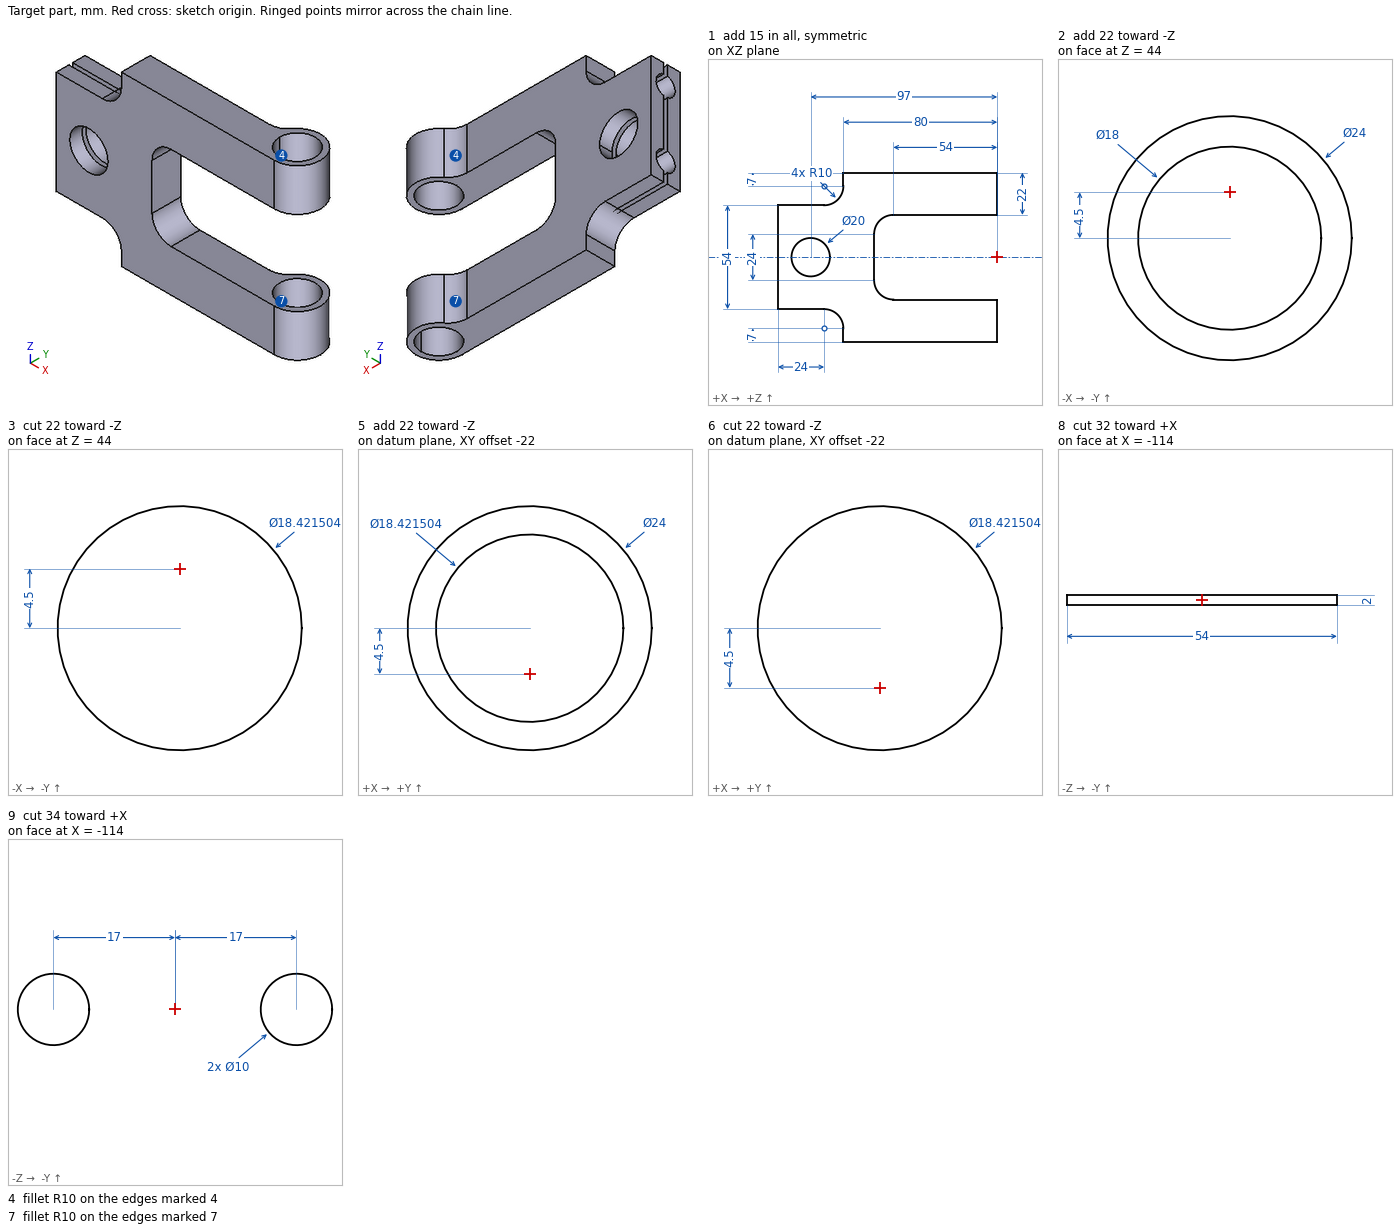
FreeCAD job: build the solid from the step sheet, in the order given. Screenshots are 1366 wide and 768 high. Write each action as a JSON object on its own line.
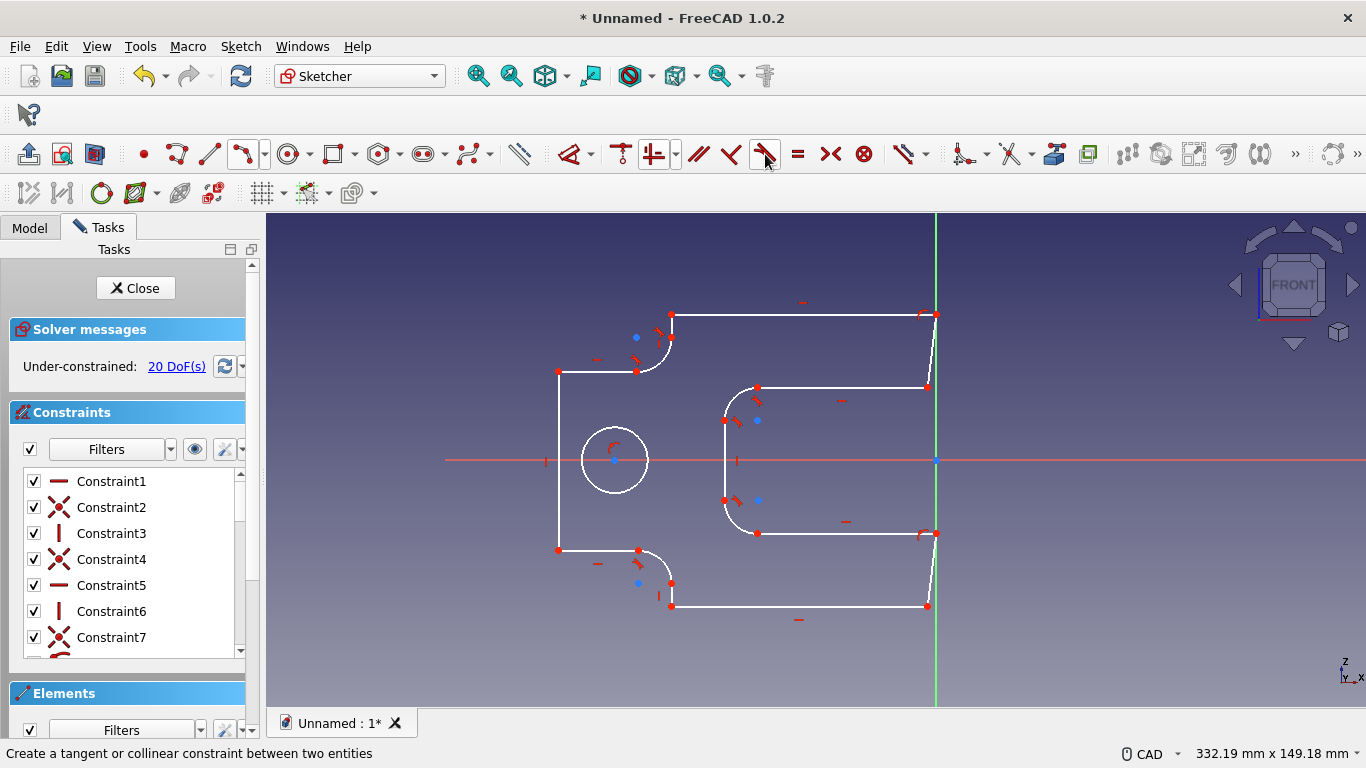
{"action": "left_click", "coordinate": [811, 534]}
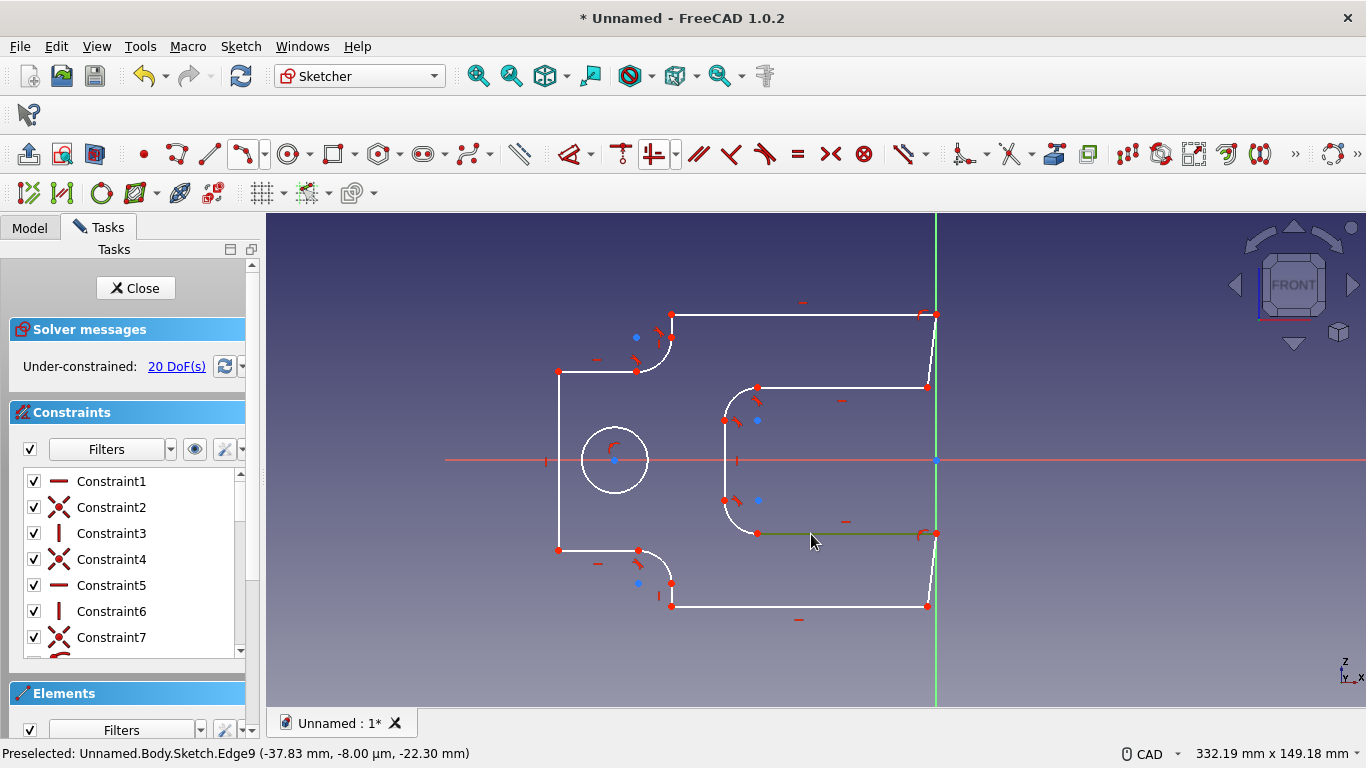
{"action": "left_click", "coordinate": [728, 515]}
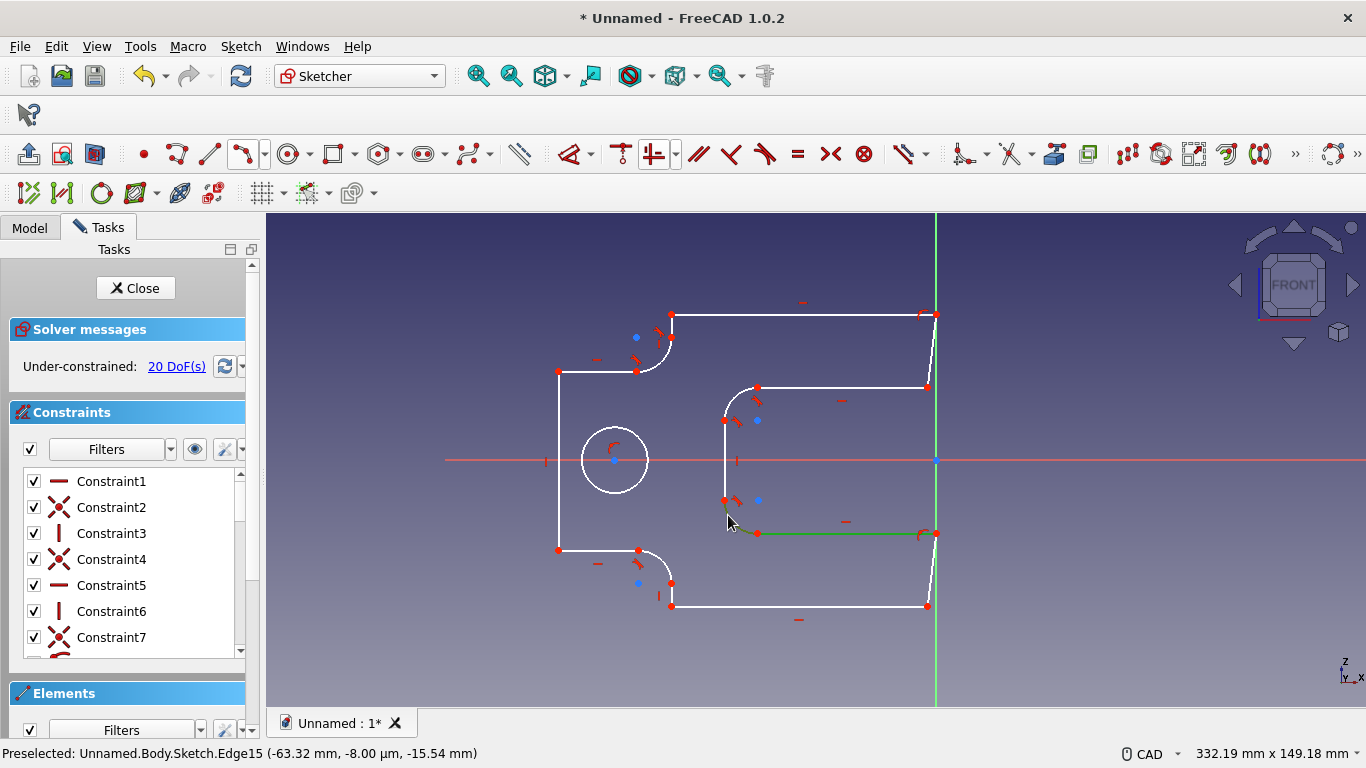
{"action": "left_click", "coordinate": [765, 154]}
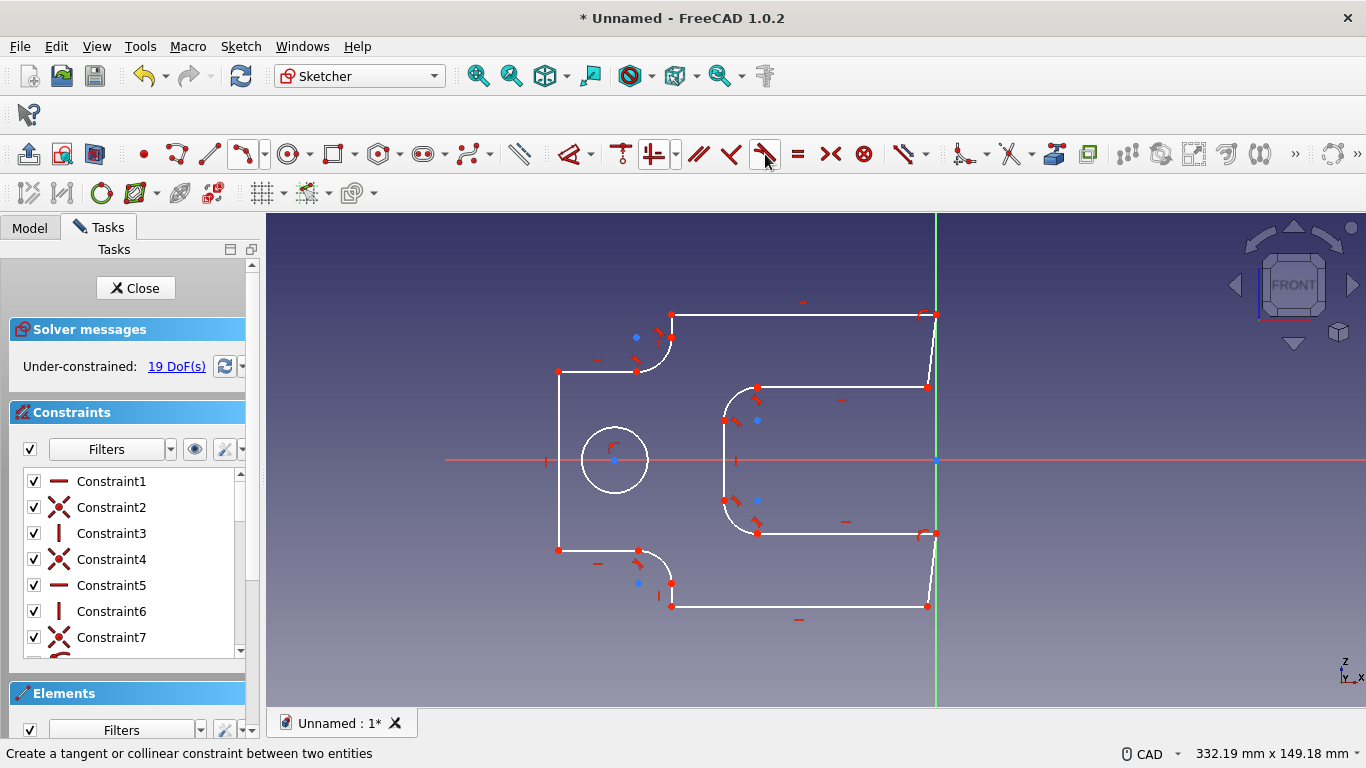
{"action": "scroll", "coordinate": [672, 598], "scroll_direction": "up", "scroll_amount": 3}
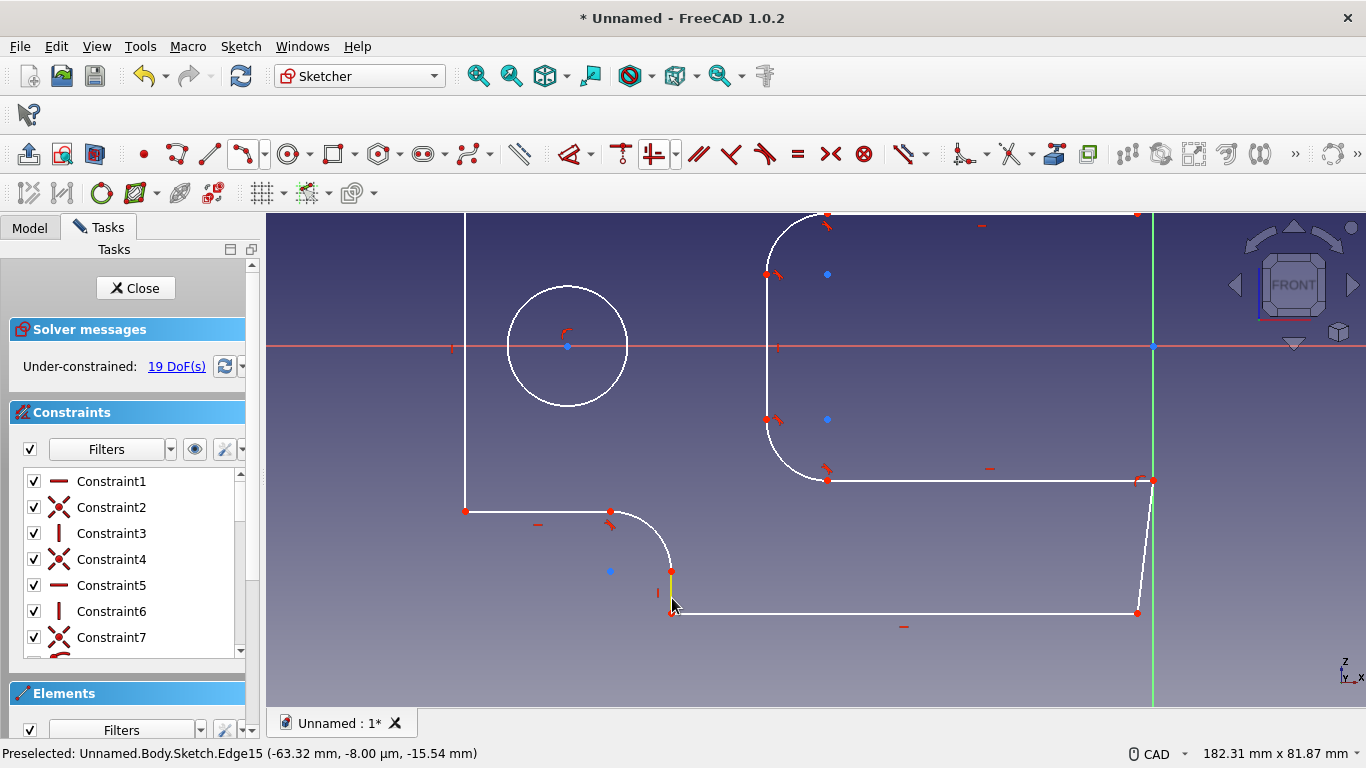
{"action": "left_click", "coordinate": [671, 597]}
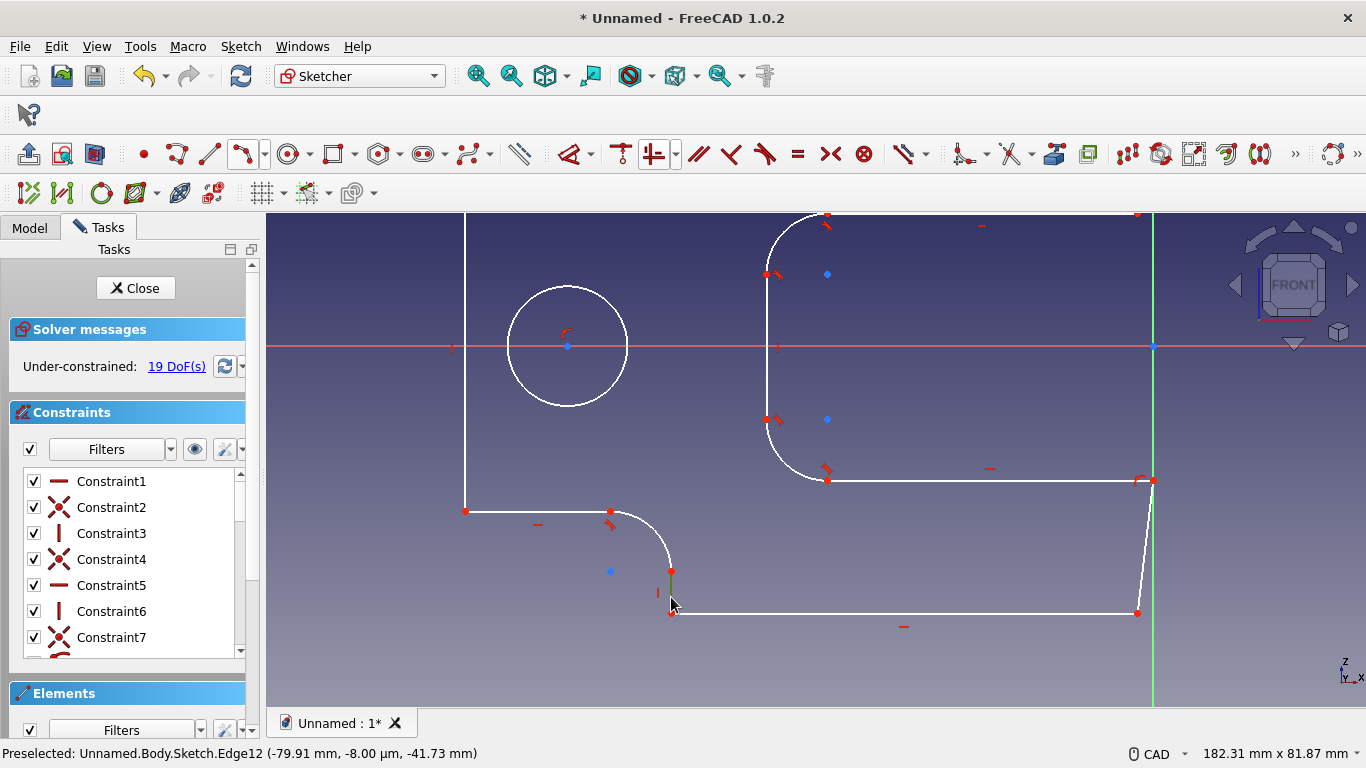
{"action": "left_click", "coordinate": [665, 545]}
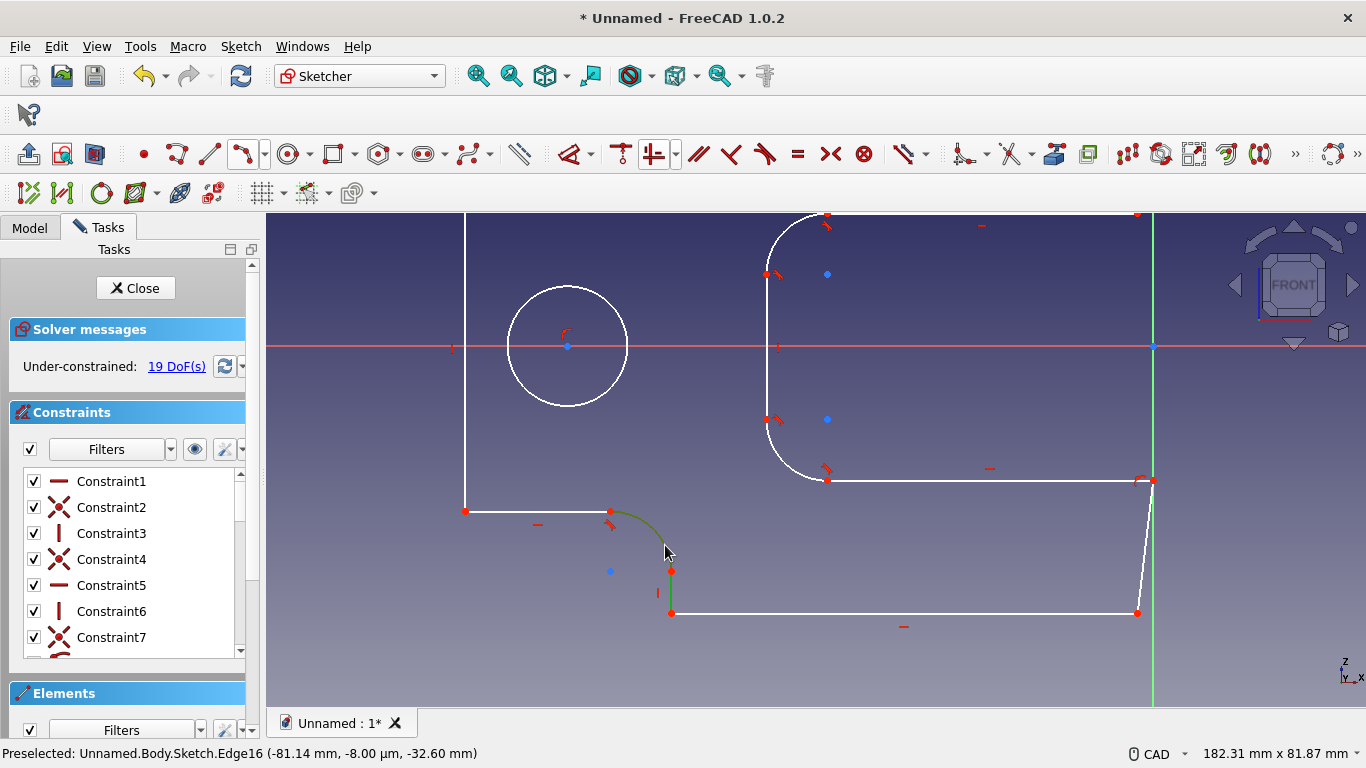
{"action": "left_click", "coordinate": [765, 154]}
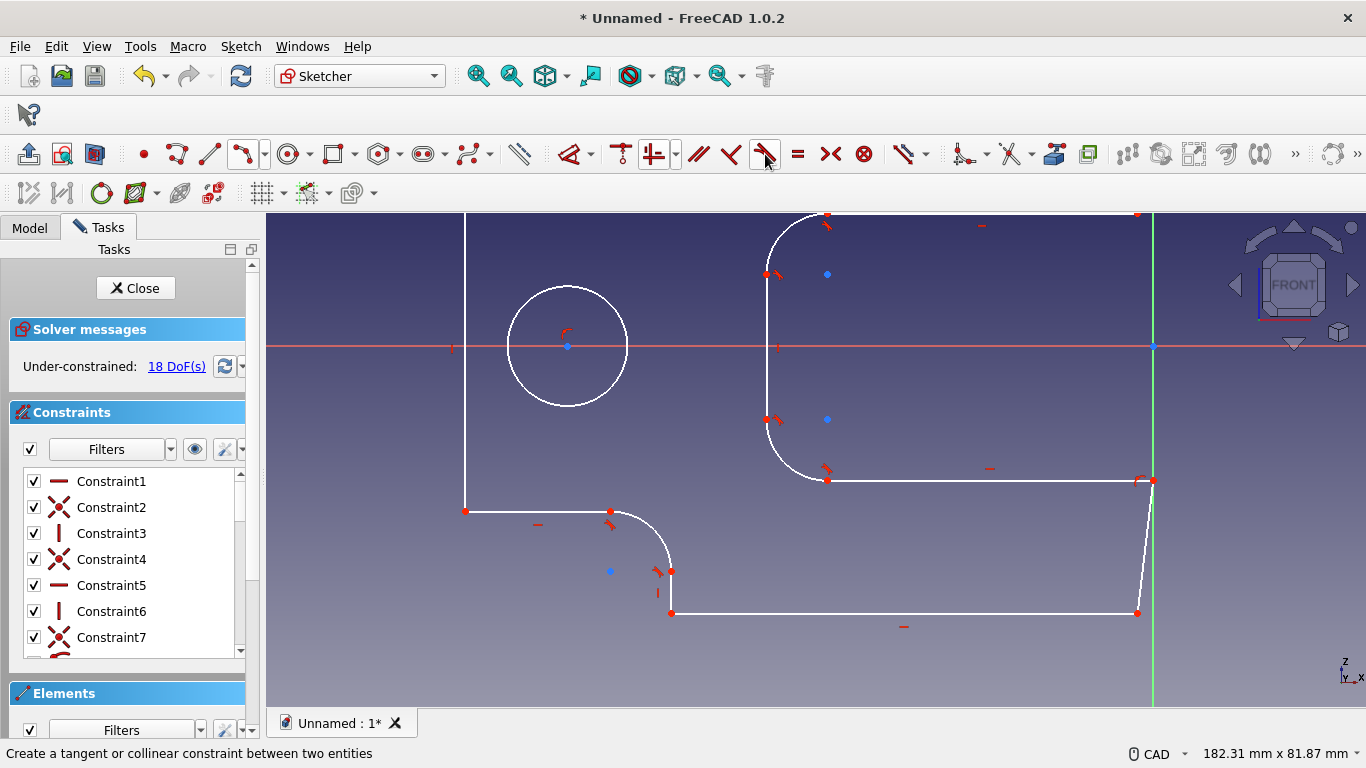
{"action": "scroll", "coordinate": [672, 598], "scroll_direction": "down", "scroll_amount": 3}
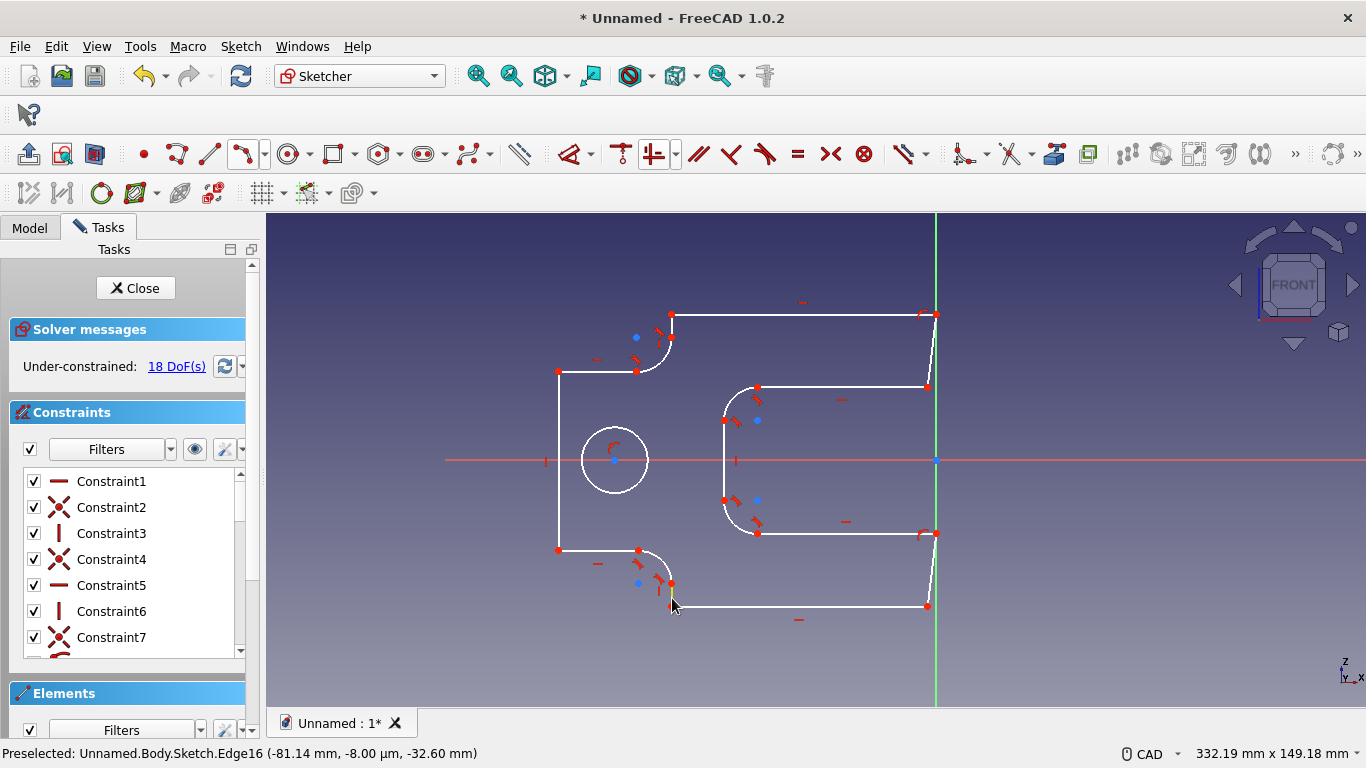
{"action": "scroll", "coordinate": [930, 366], "scroll_direction": "up", "scroll_amount": 5}